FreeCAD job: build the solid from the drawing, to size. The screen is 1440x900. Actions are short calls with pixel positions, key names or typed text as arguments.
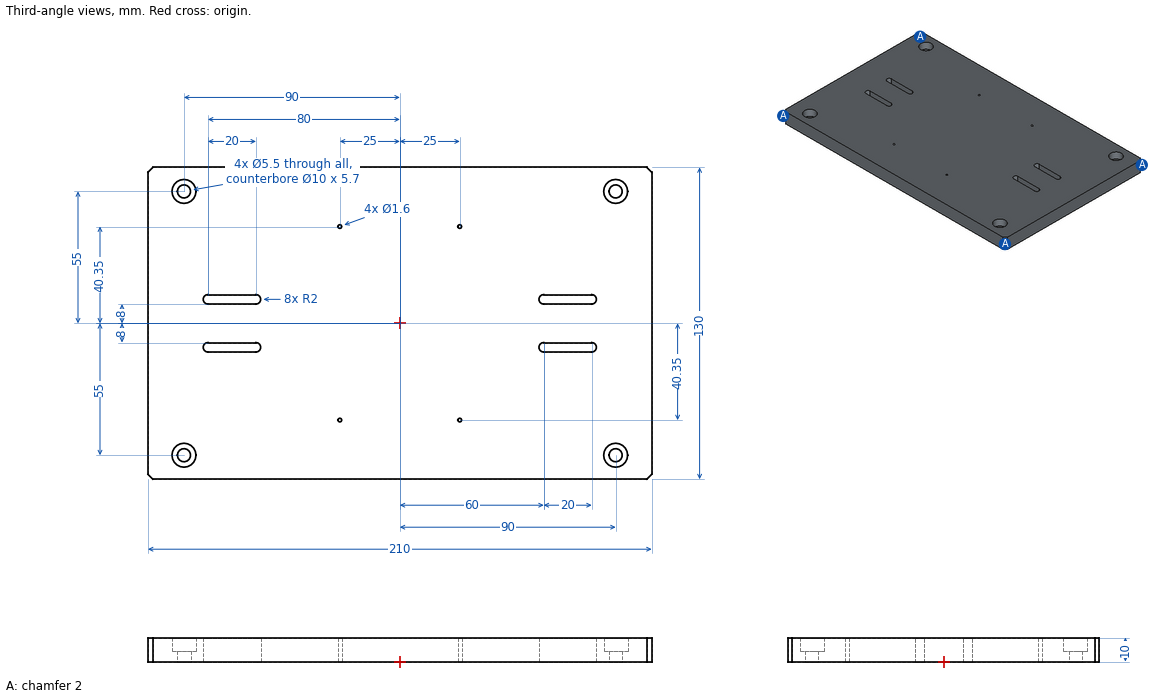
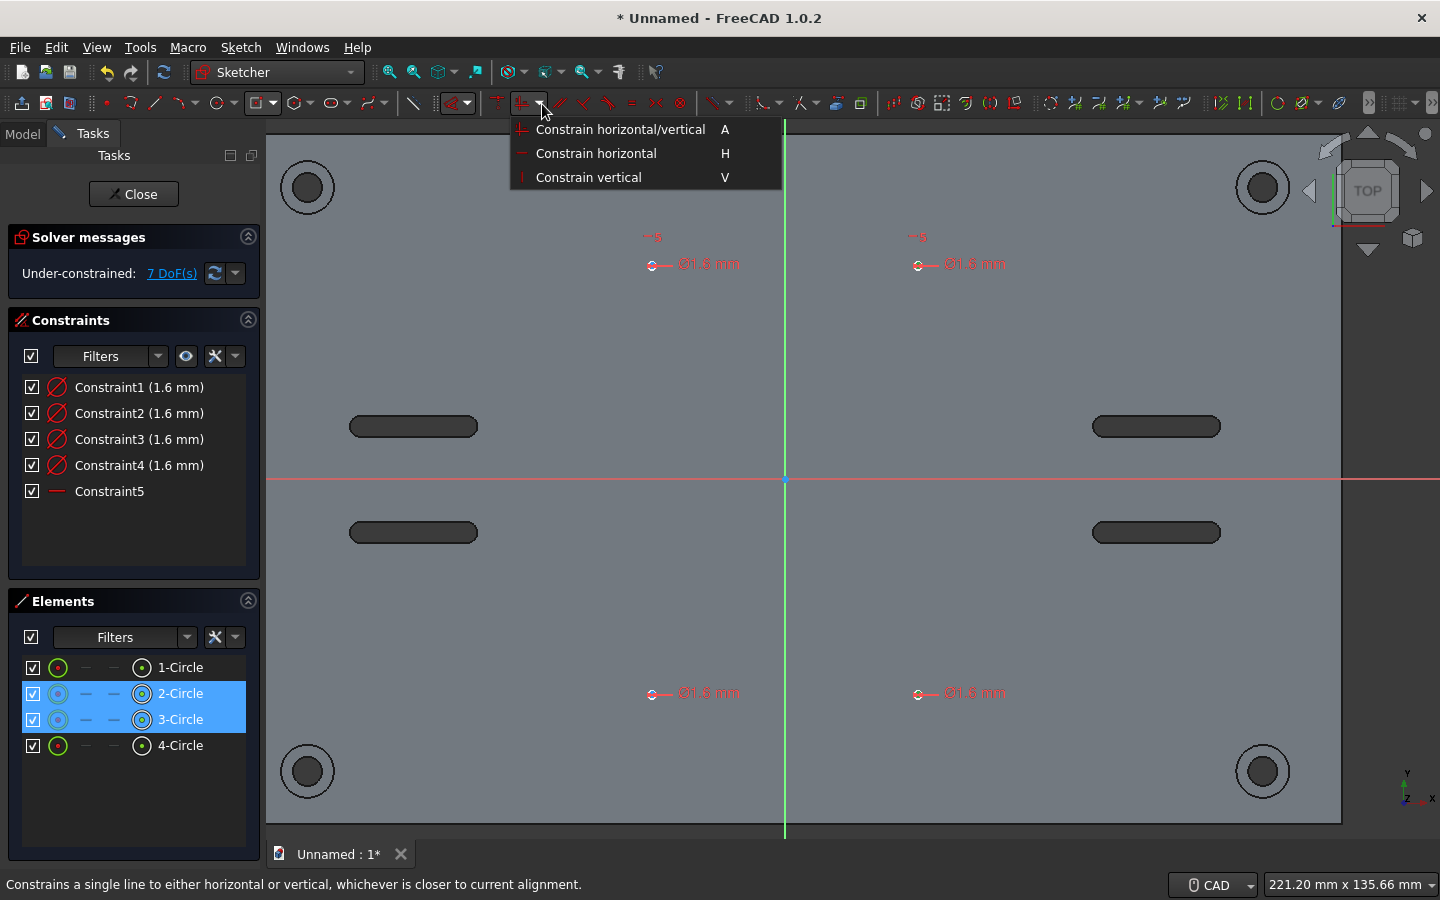
click(646, 177)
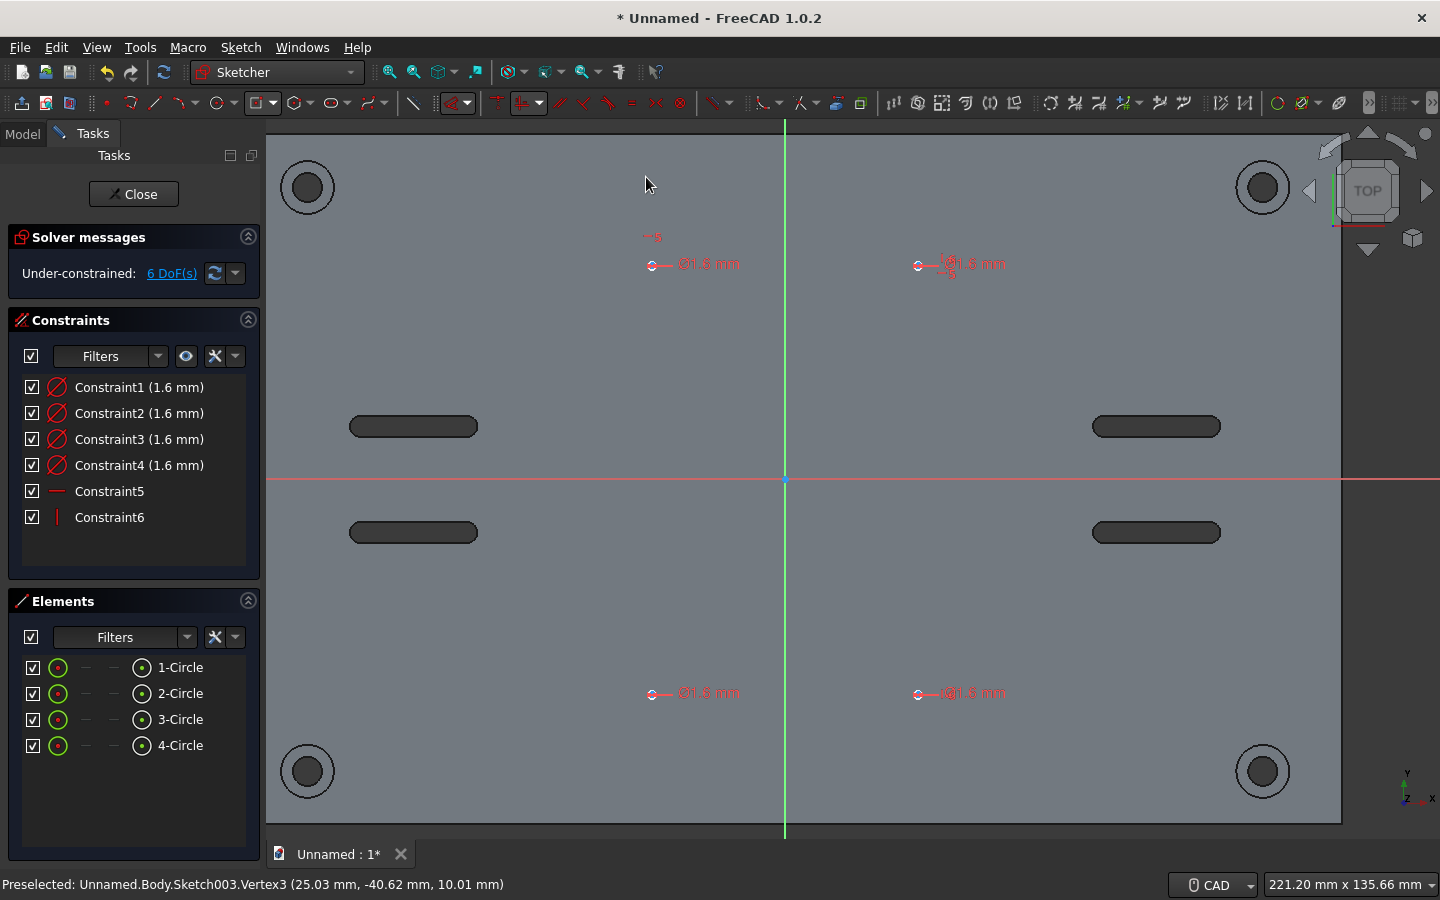
click(652, 266)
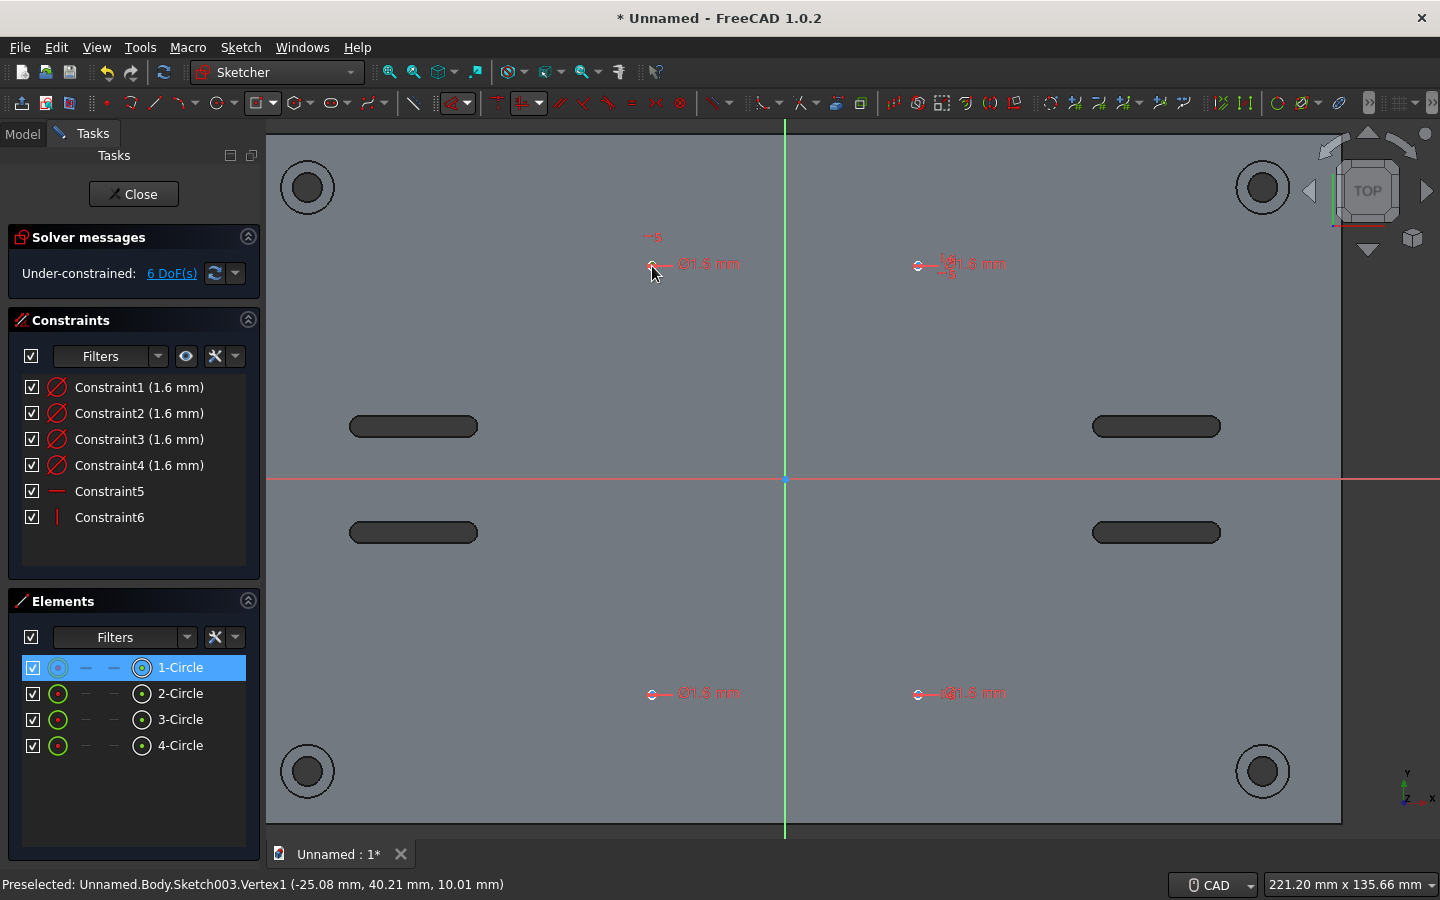
click(652, 695)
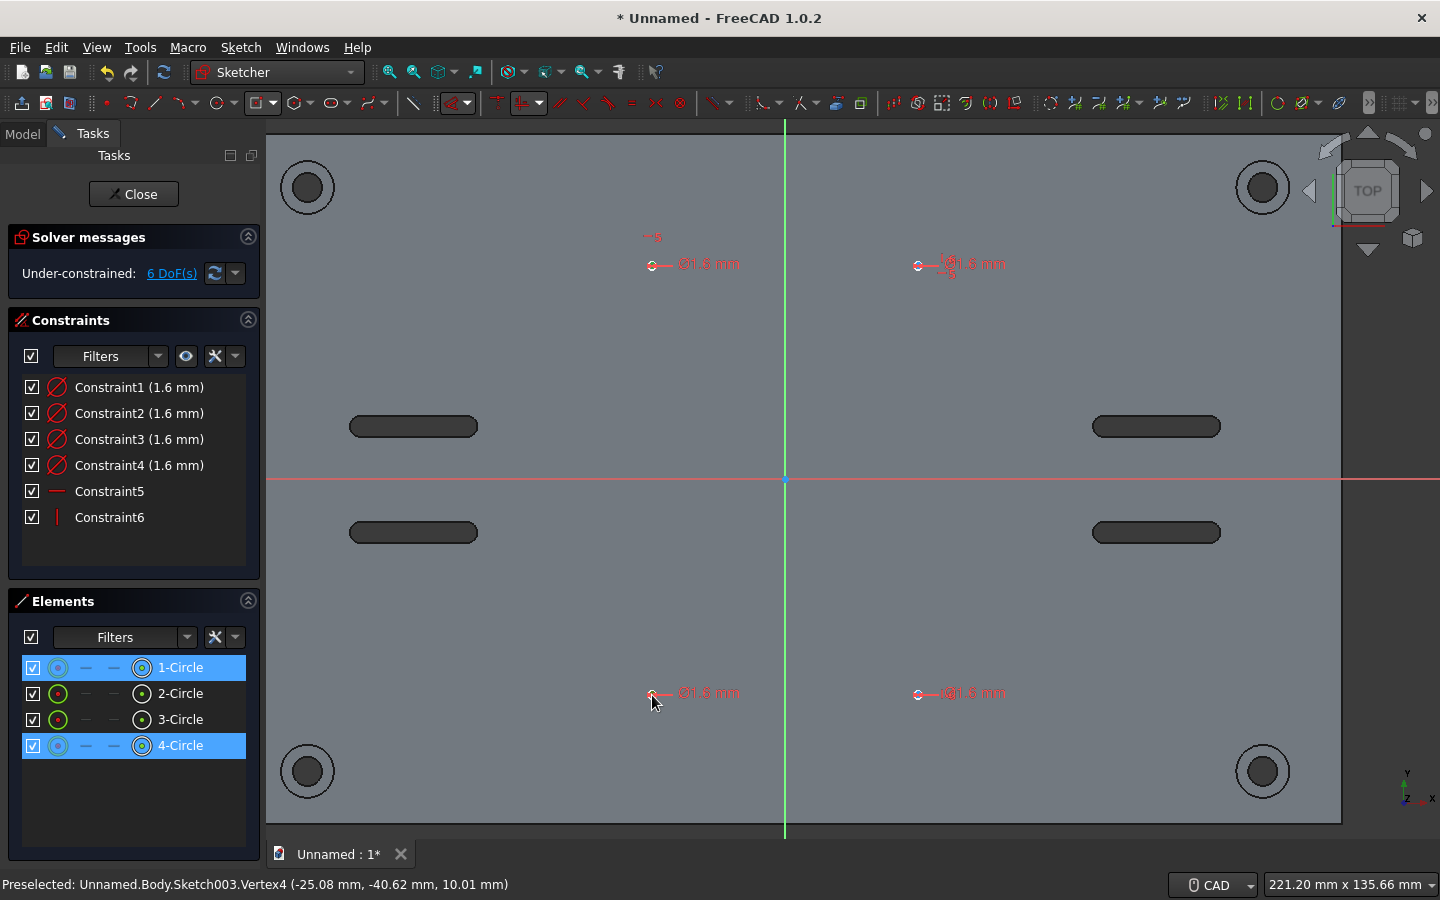
click(542, 104)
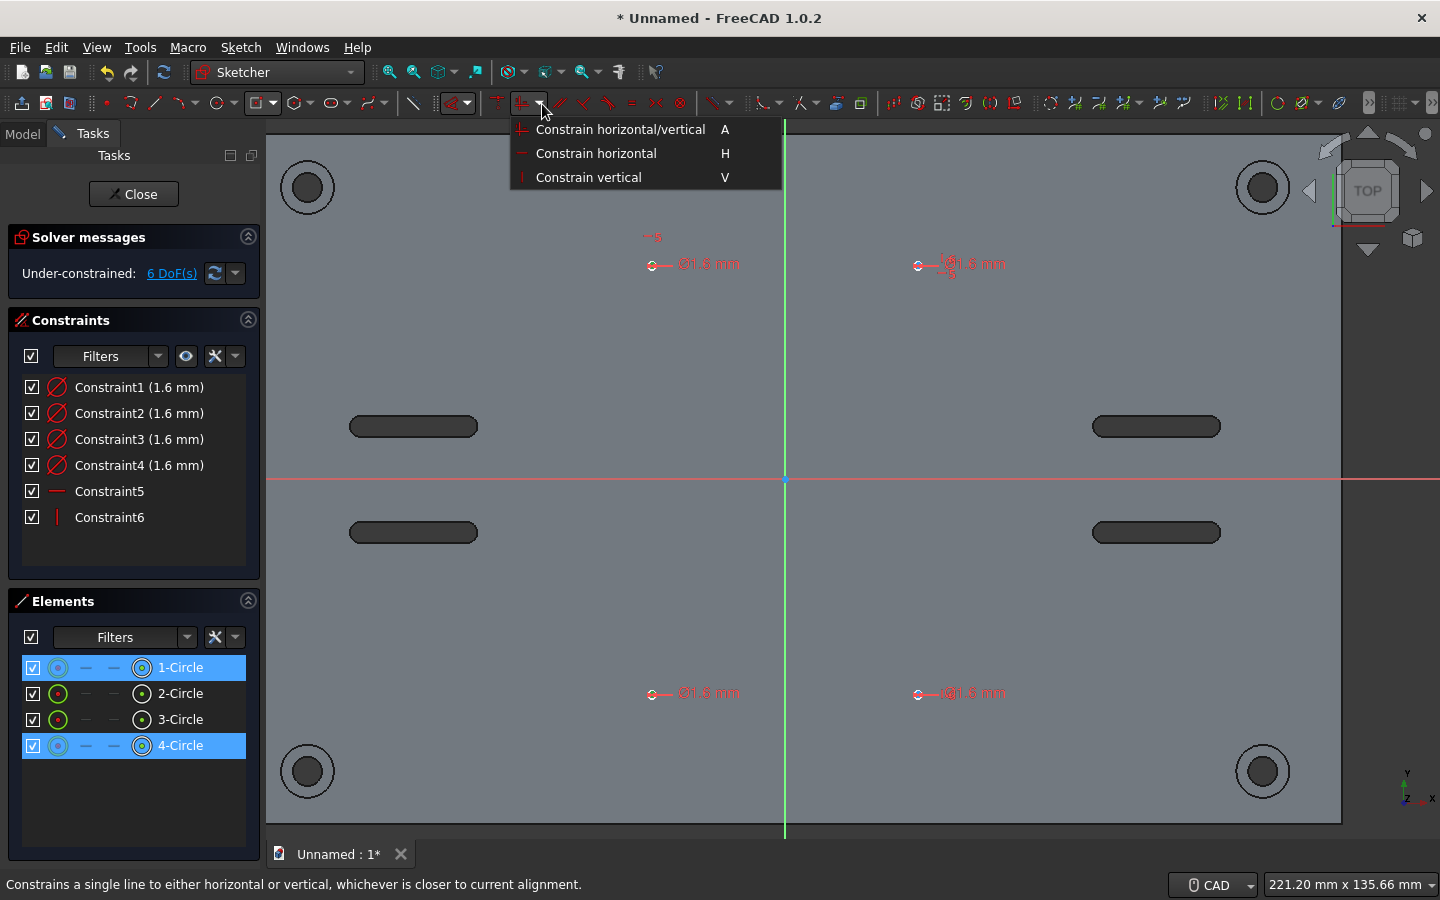
click(646, 177)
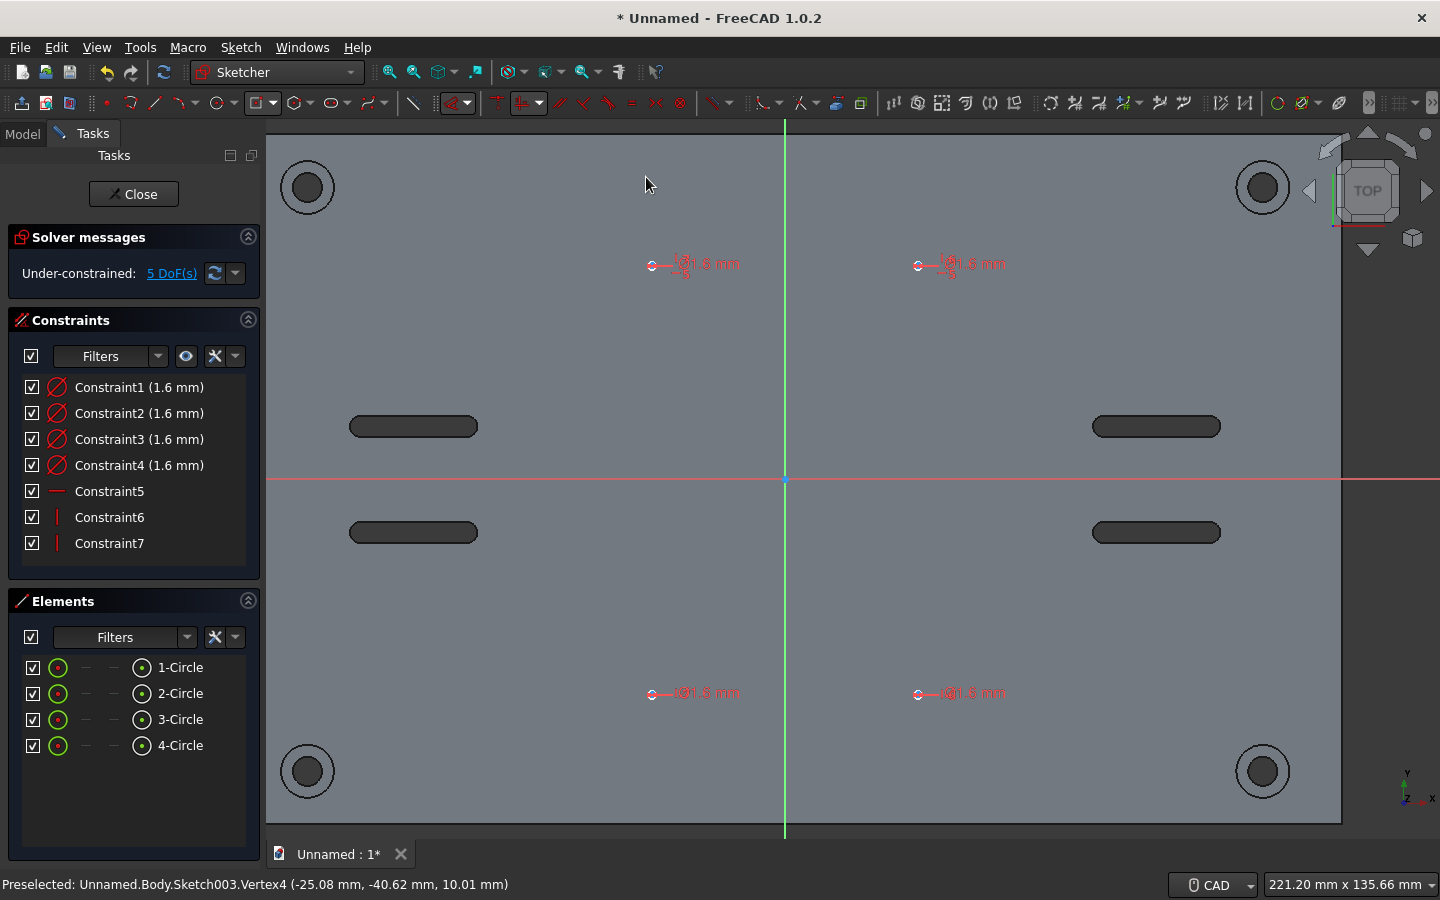
click(918, 695)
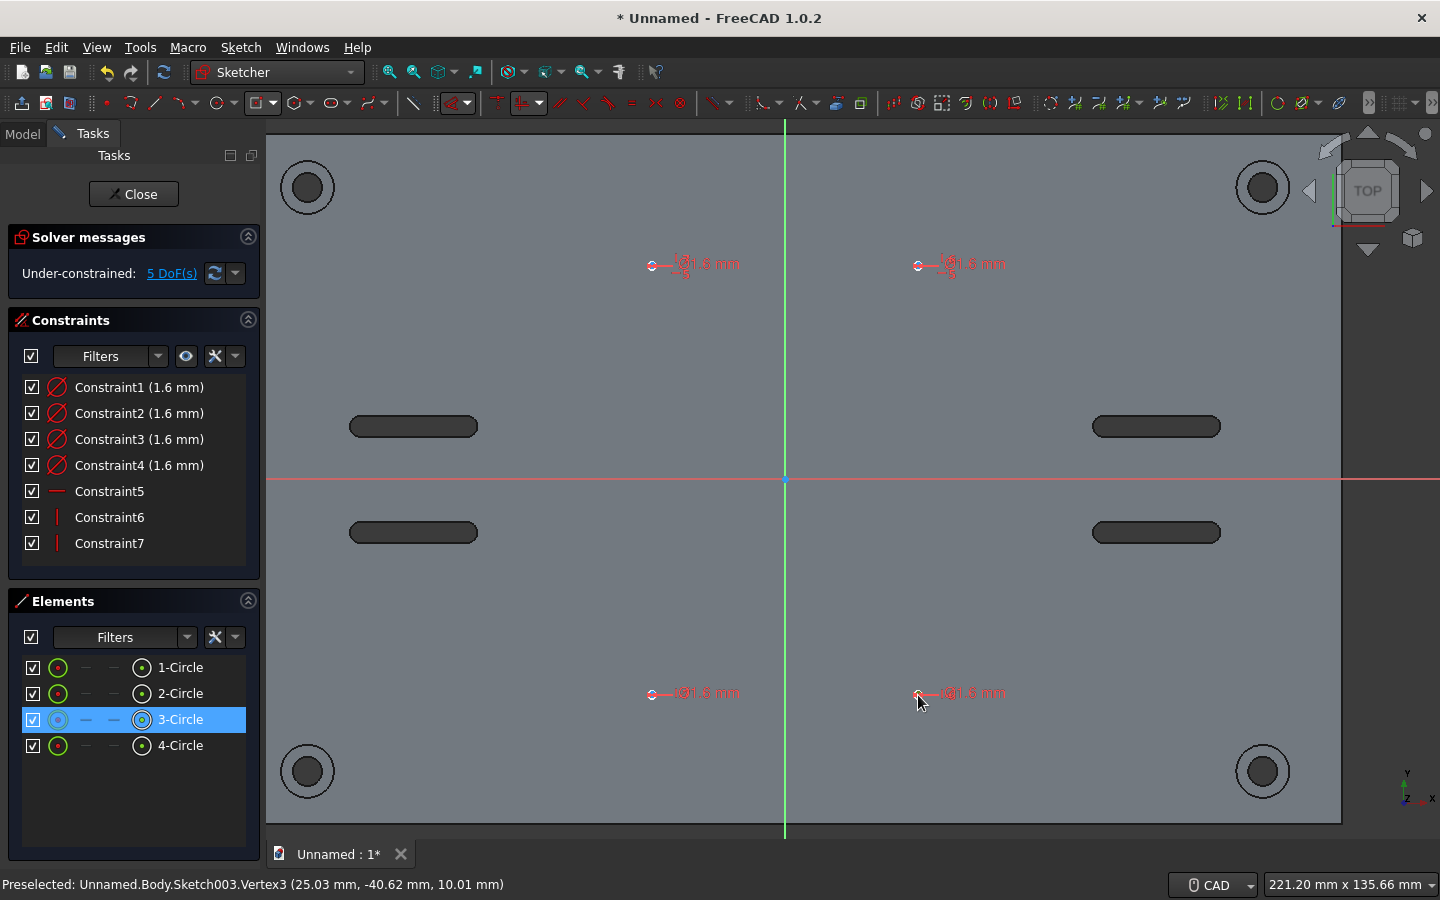
click(652, 695)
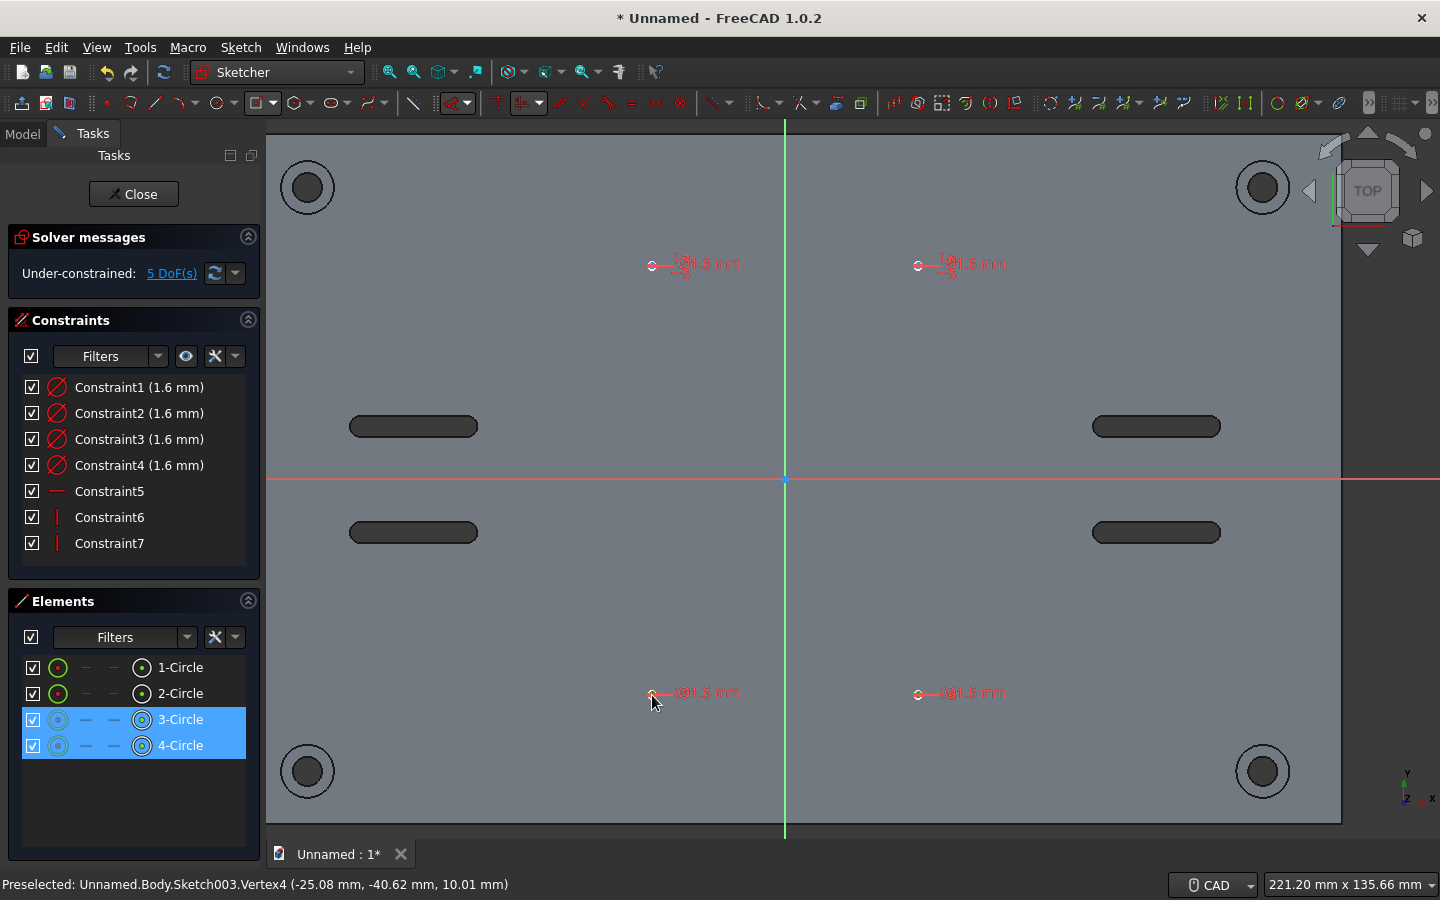
key(h)